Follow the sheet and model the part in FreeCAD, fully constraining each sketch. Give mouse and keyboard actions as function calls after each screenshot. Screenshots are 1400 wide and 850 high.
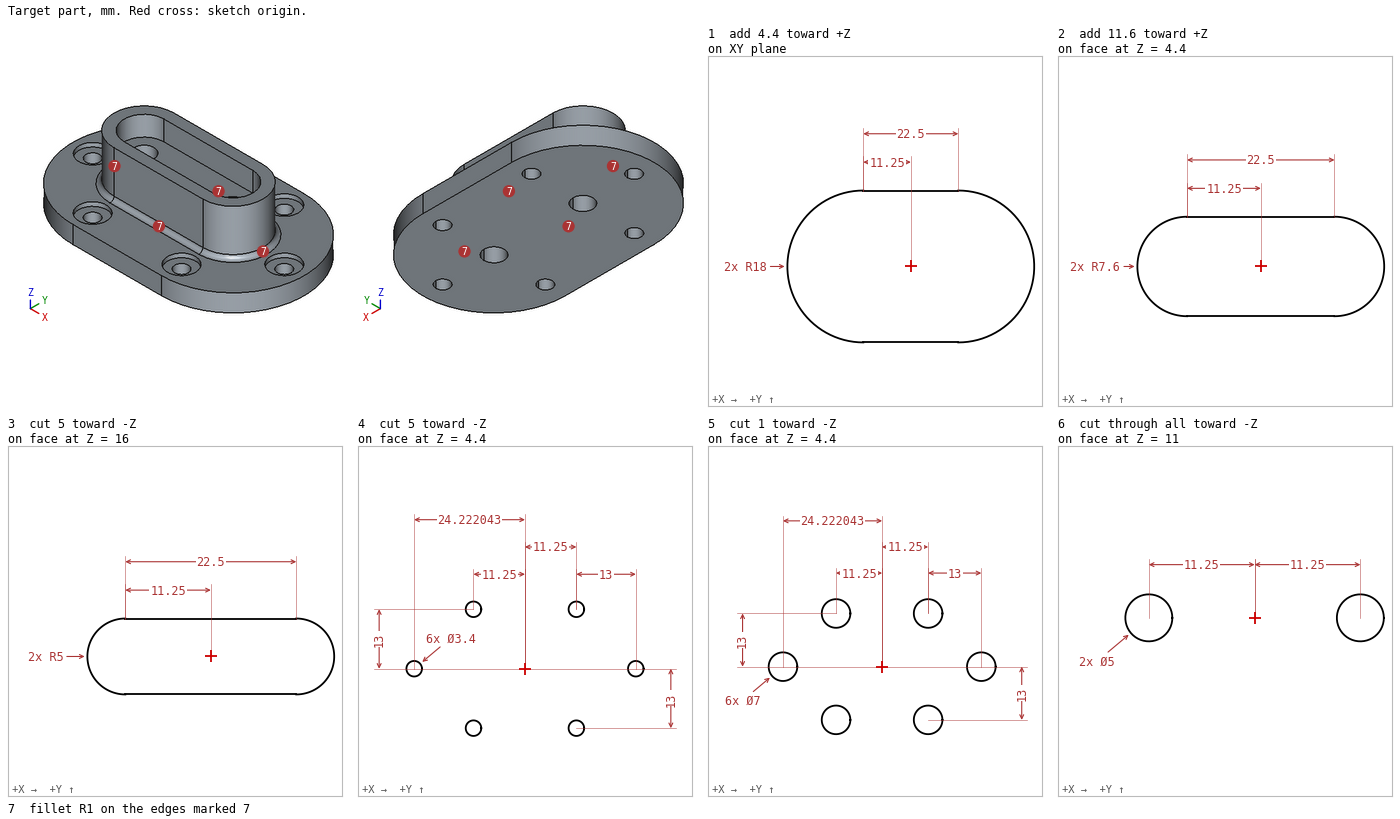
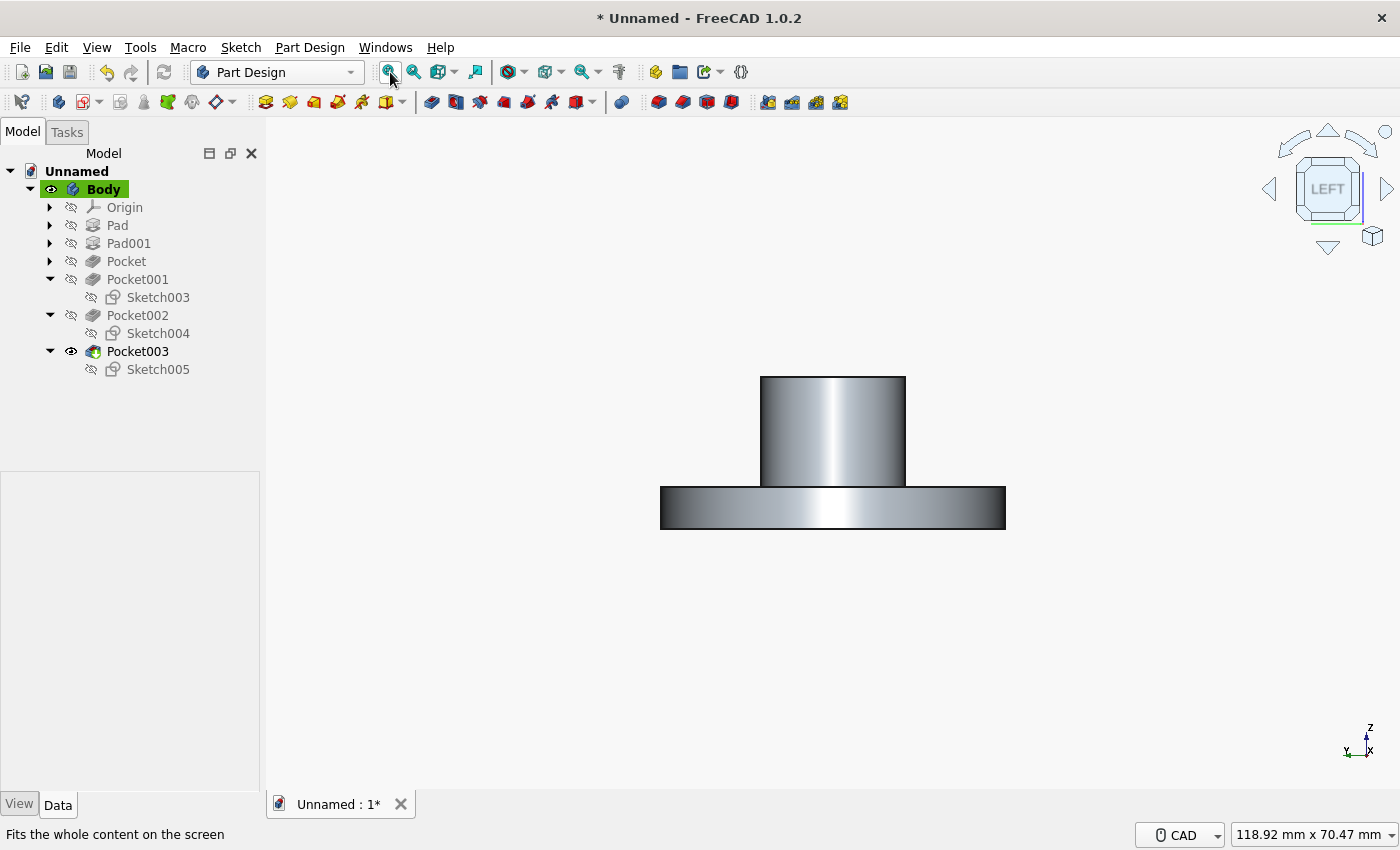
key(v)
key(3)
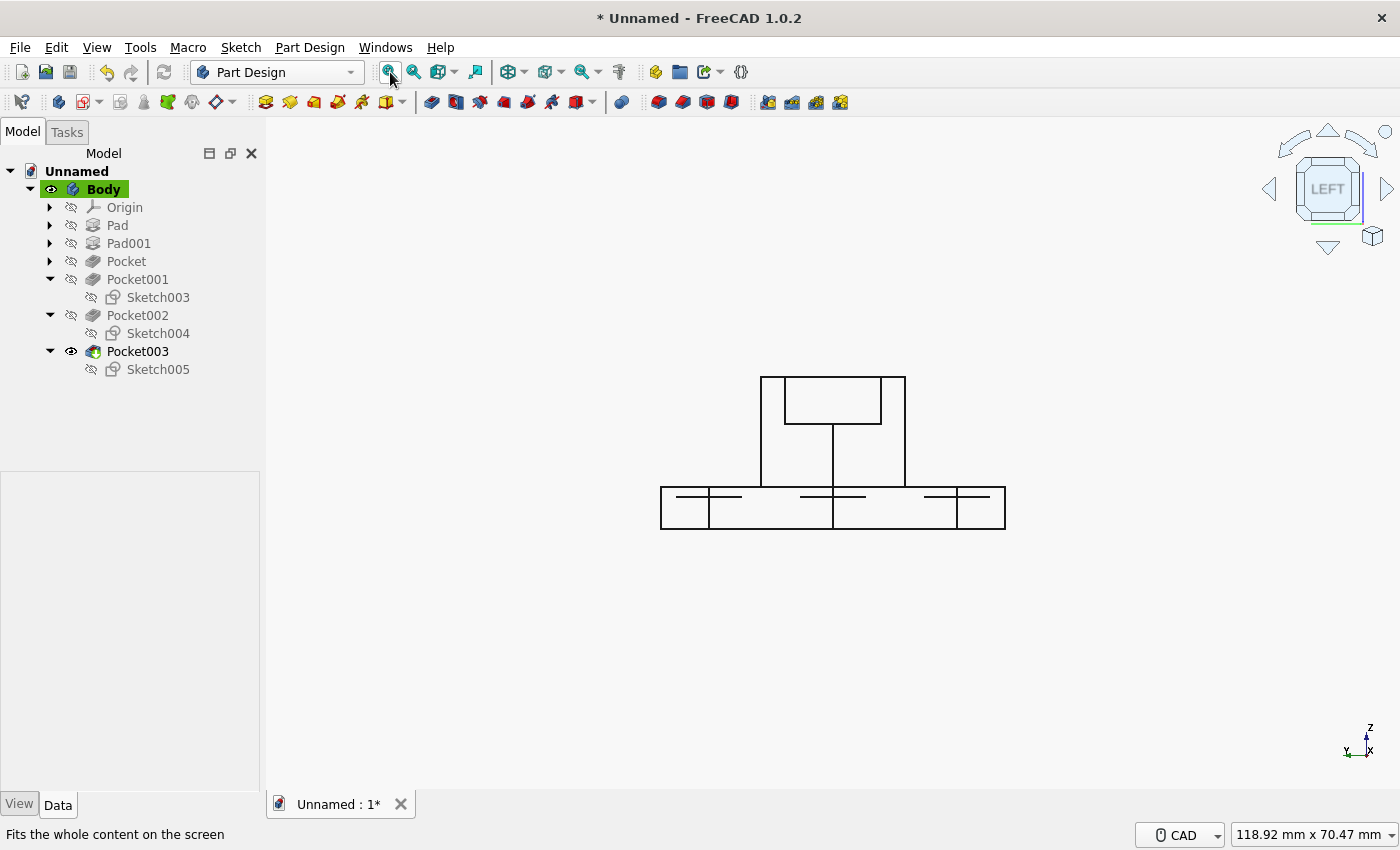
key(0)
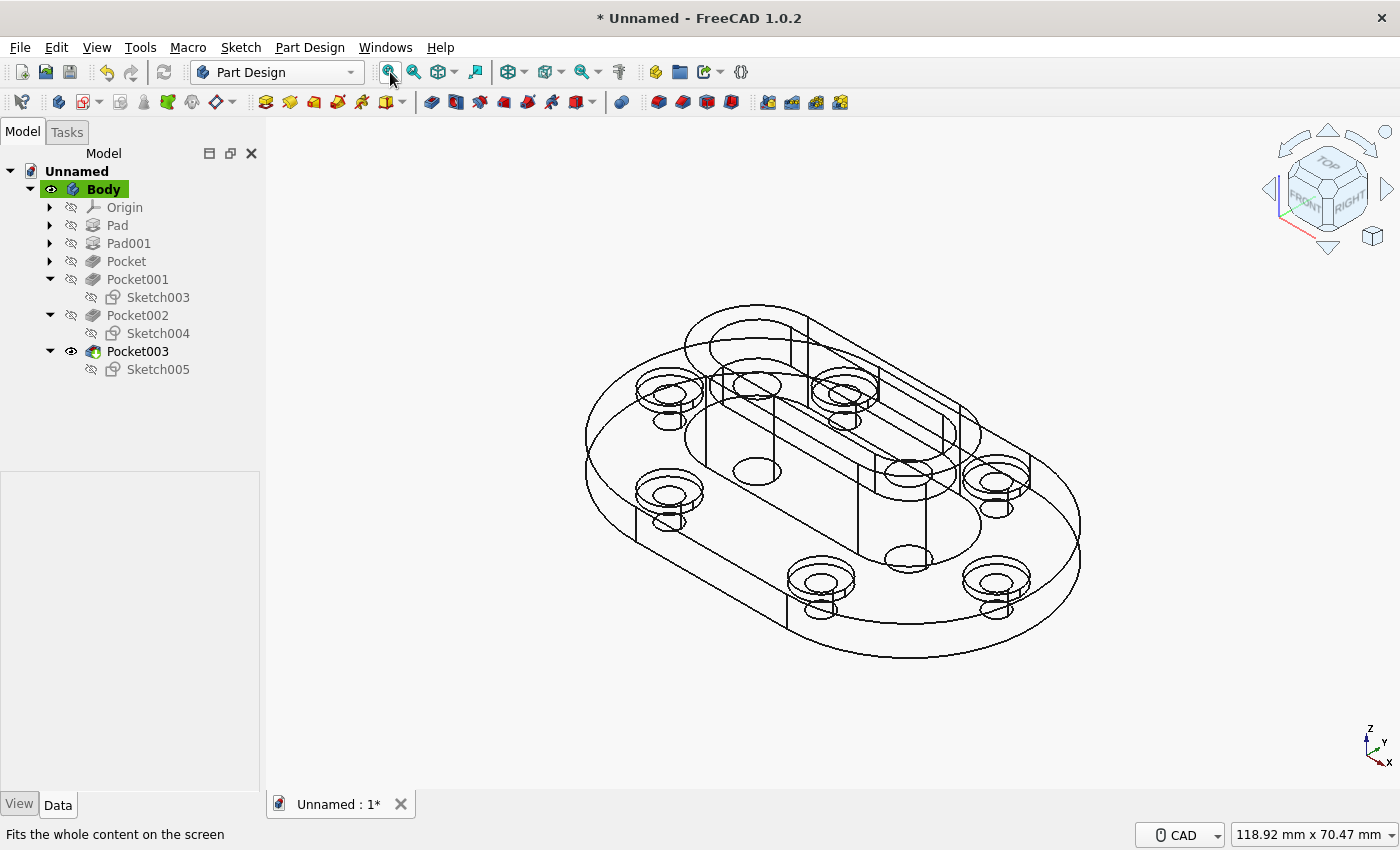
click(693, 417)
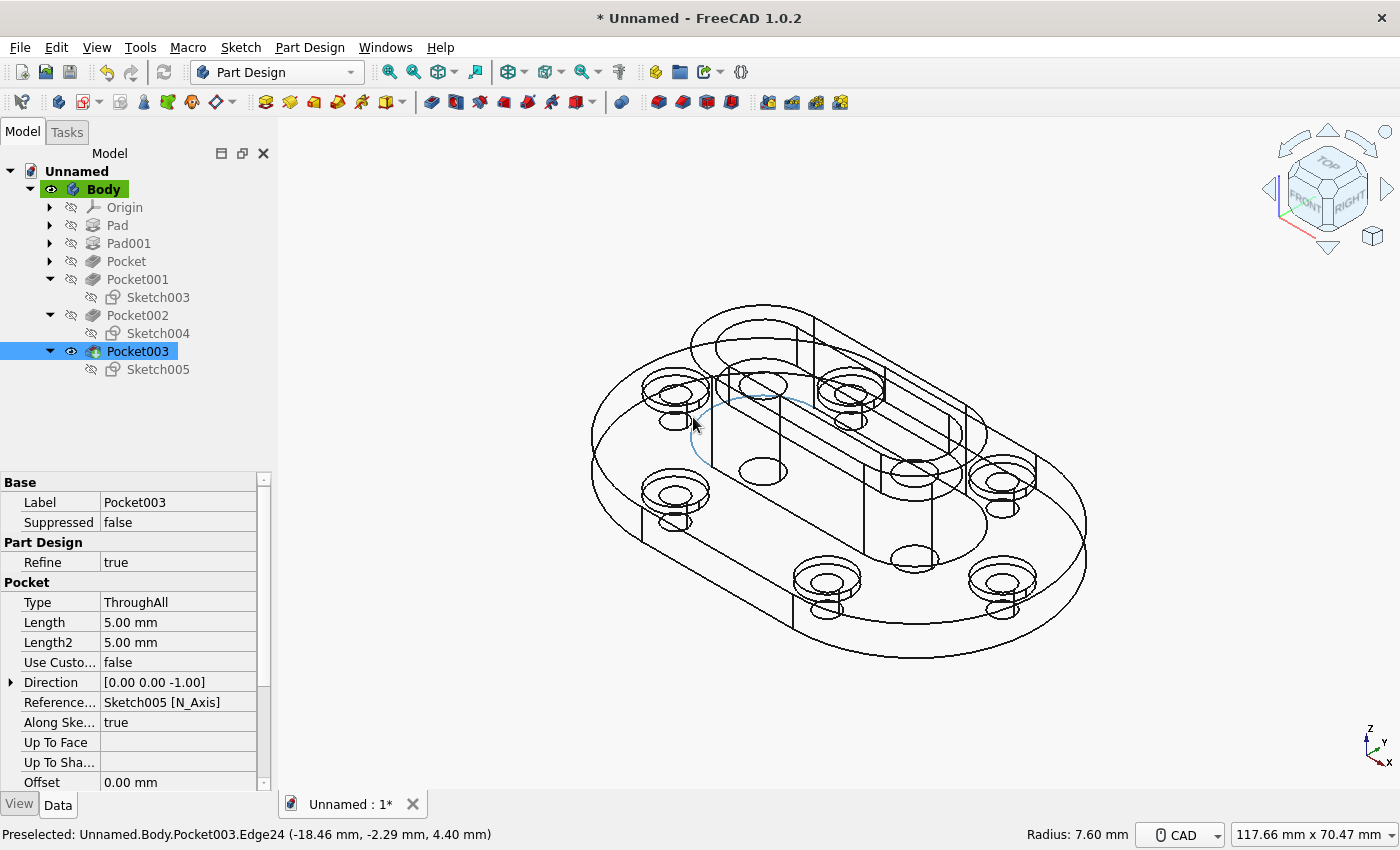
click(788, 510, ctrl)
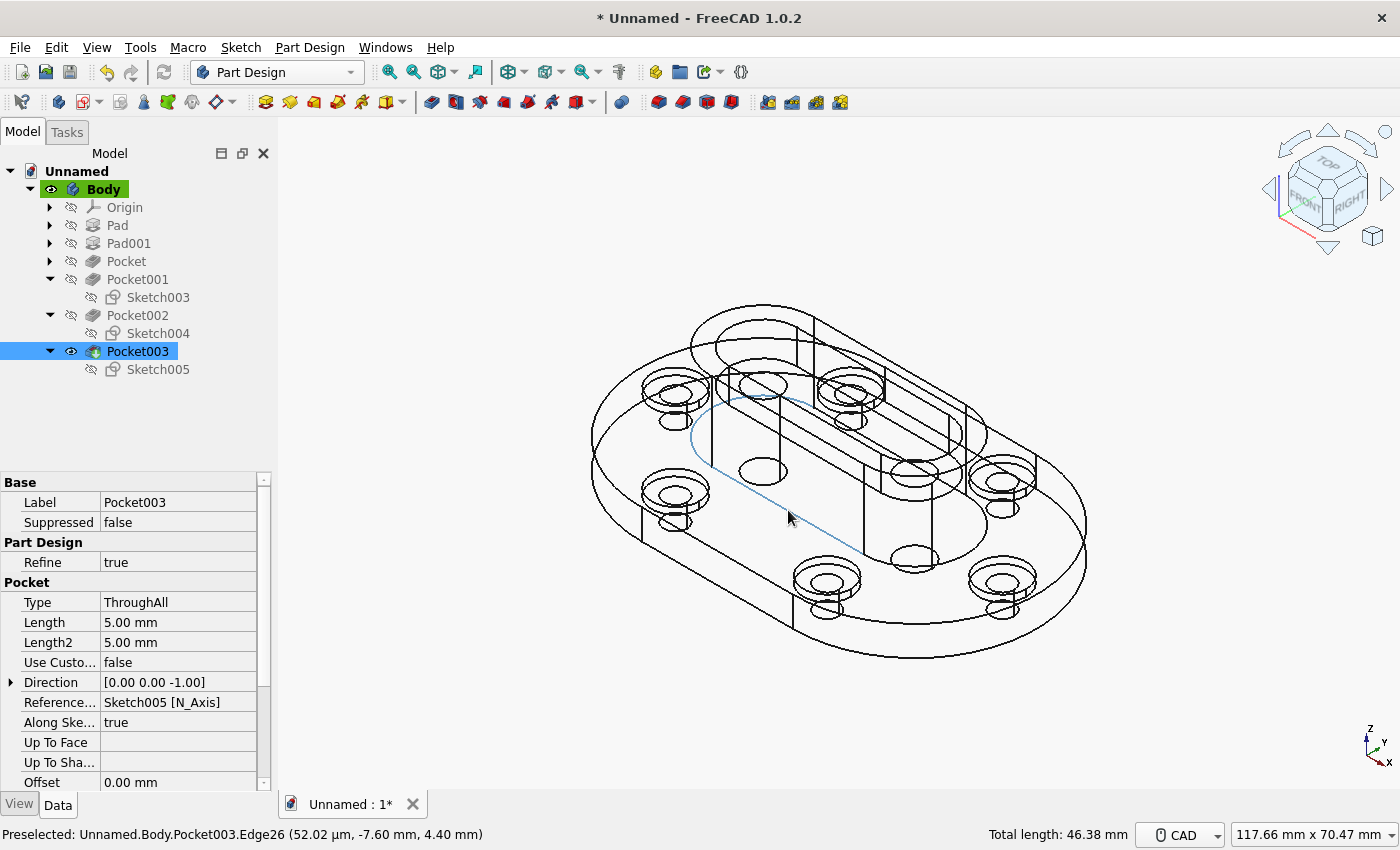
click(966, 553, ctrl)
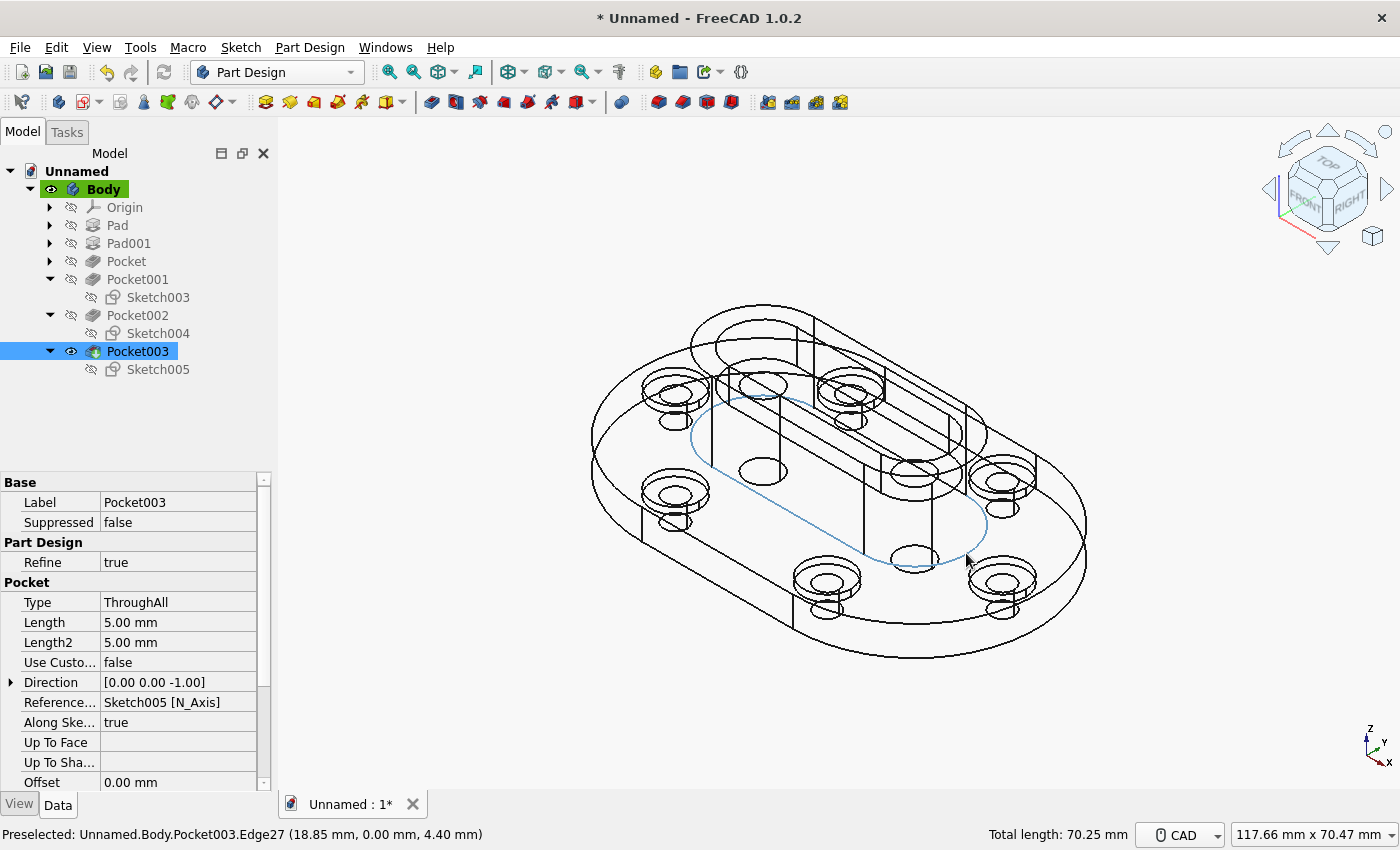
click(890, 450, ctrl)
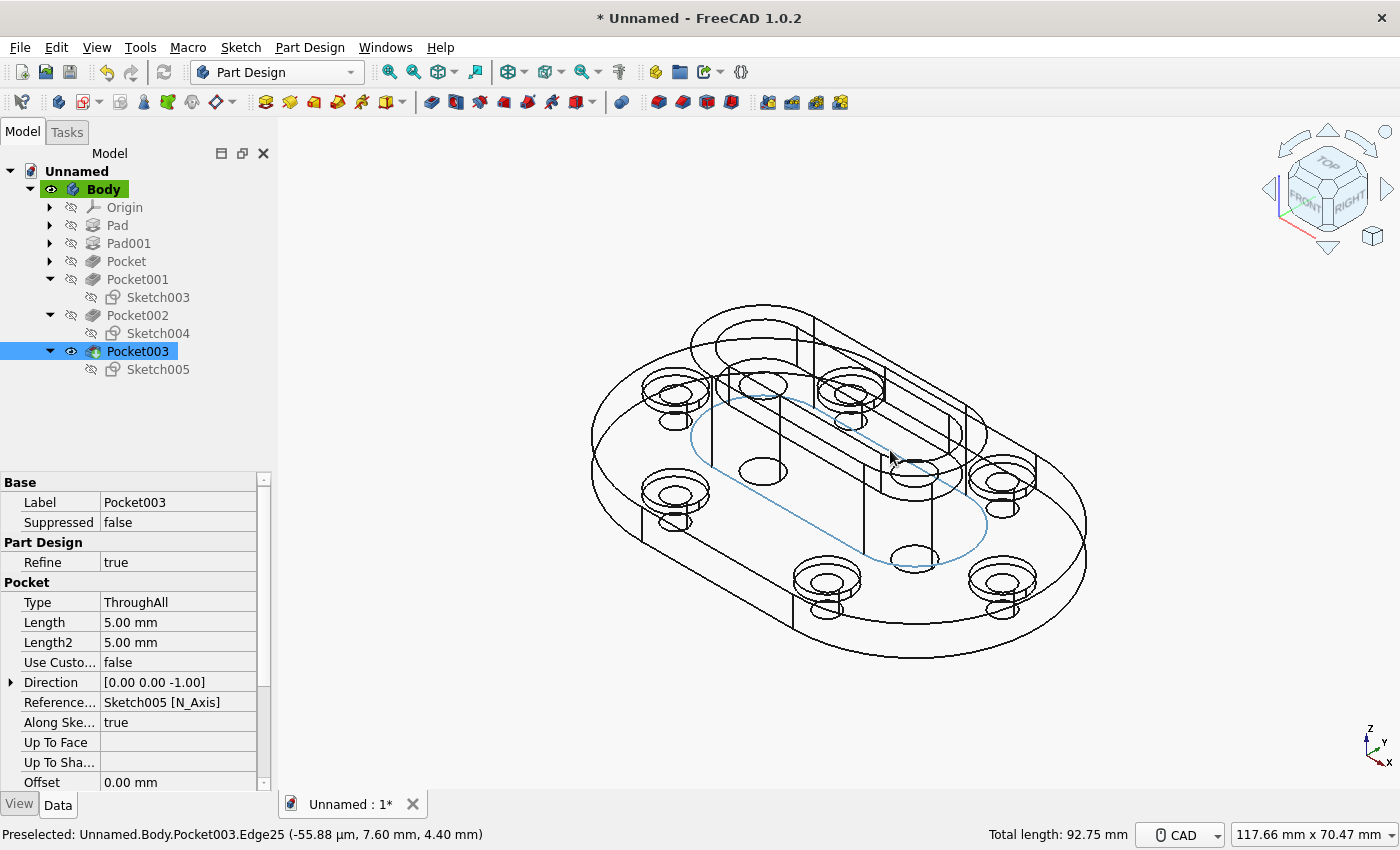
key(v)
key(1)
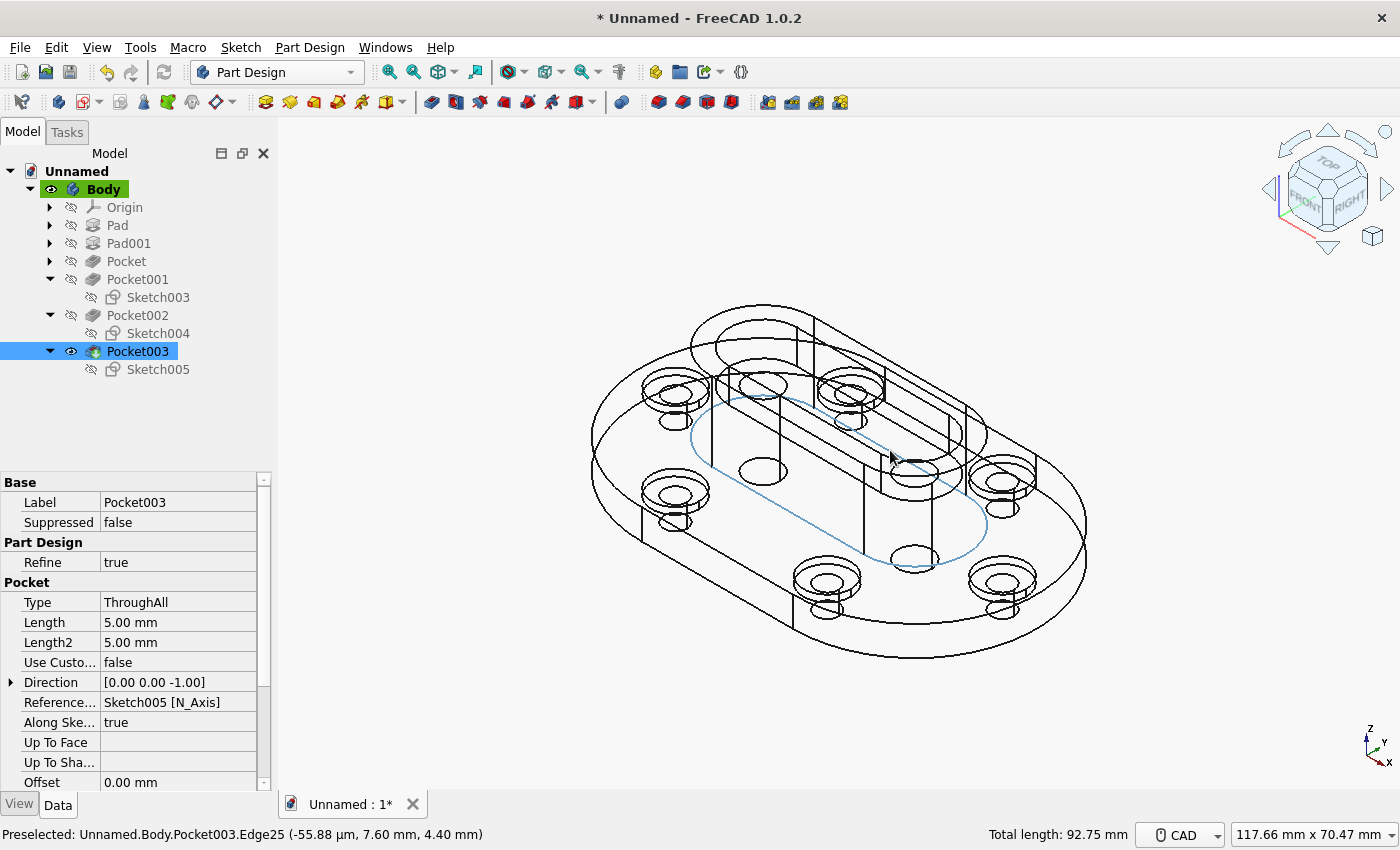
click(660, 102)